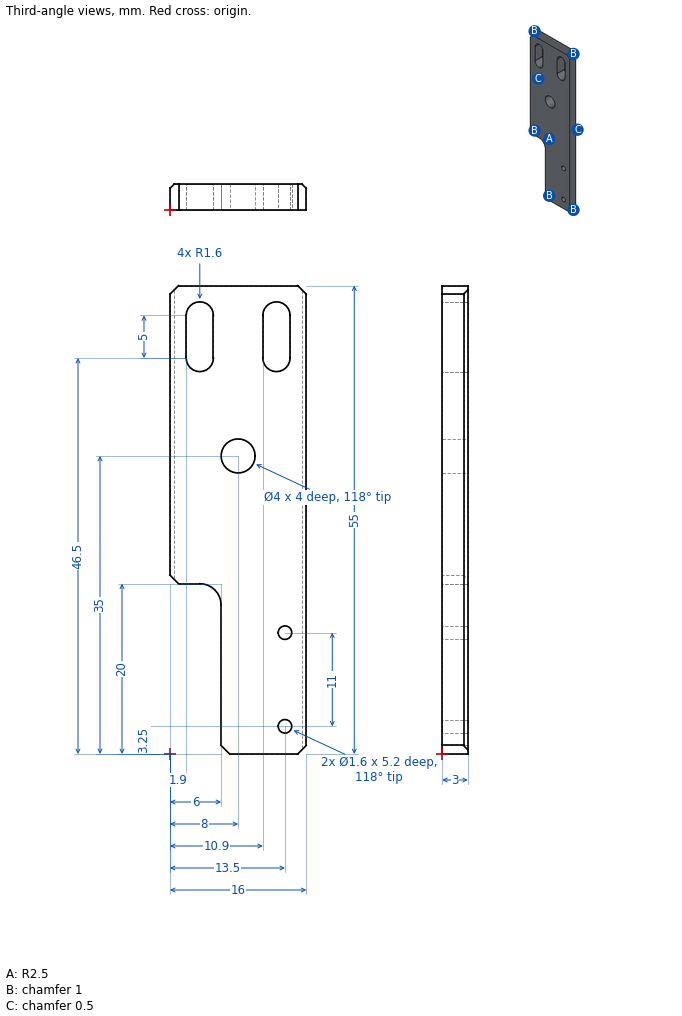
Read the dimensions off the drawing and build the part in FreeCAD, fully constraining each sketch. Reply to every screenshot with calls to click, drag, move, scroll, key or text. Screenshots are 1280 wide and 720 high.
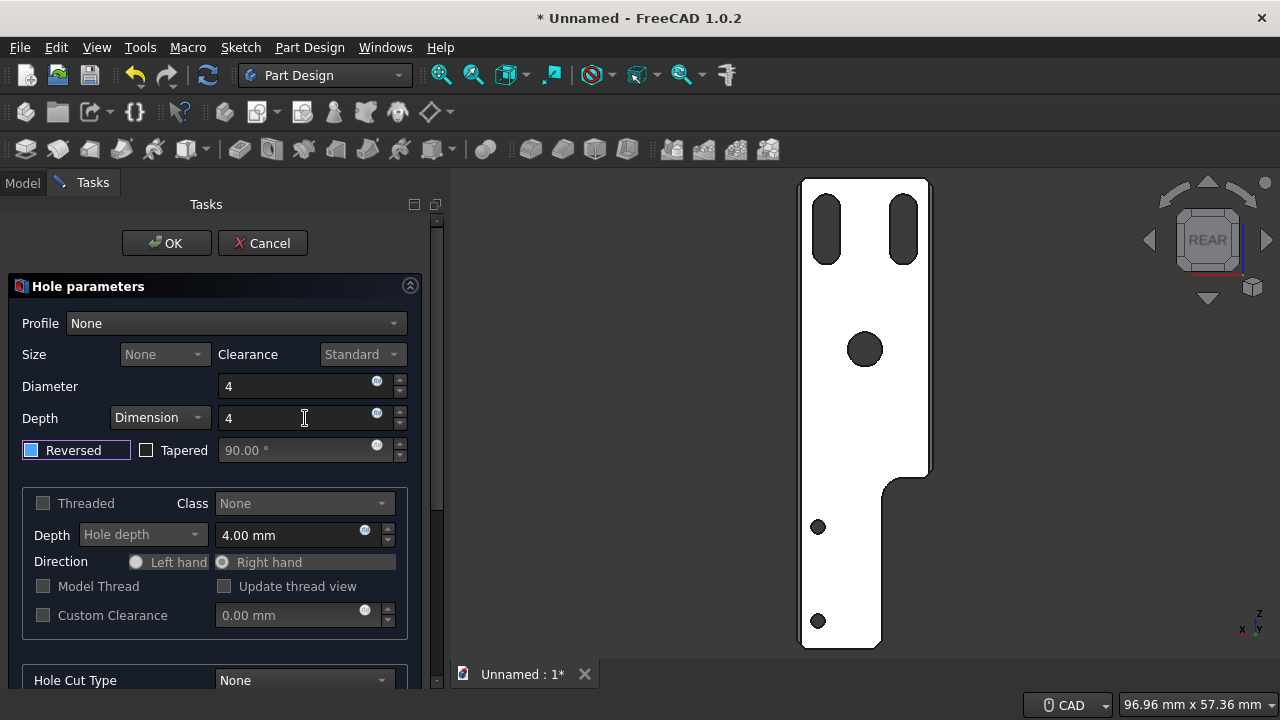
click(167, 243)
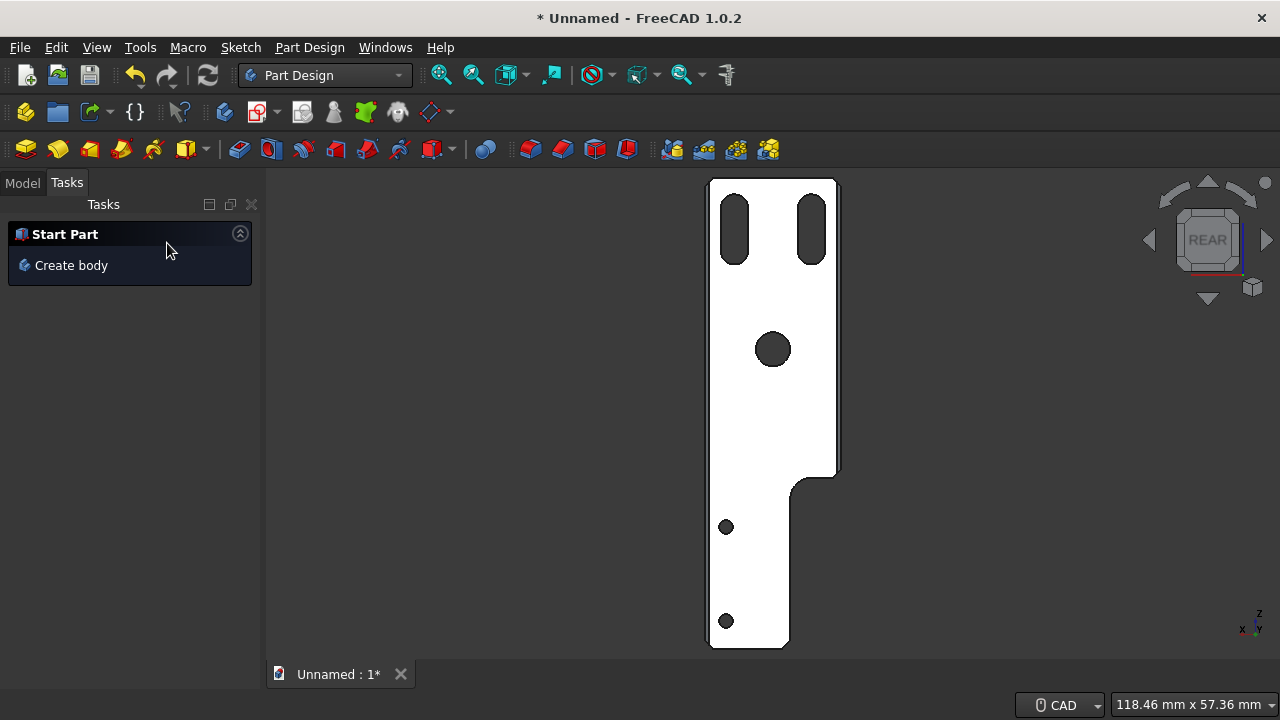
key(0)